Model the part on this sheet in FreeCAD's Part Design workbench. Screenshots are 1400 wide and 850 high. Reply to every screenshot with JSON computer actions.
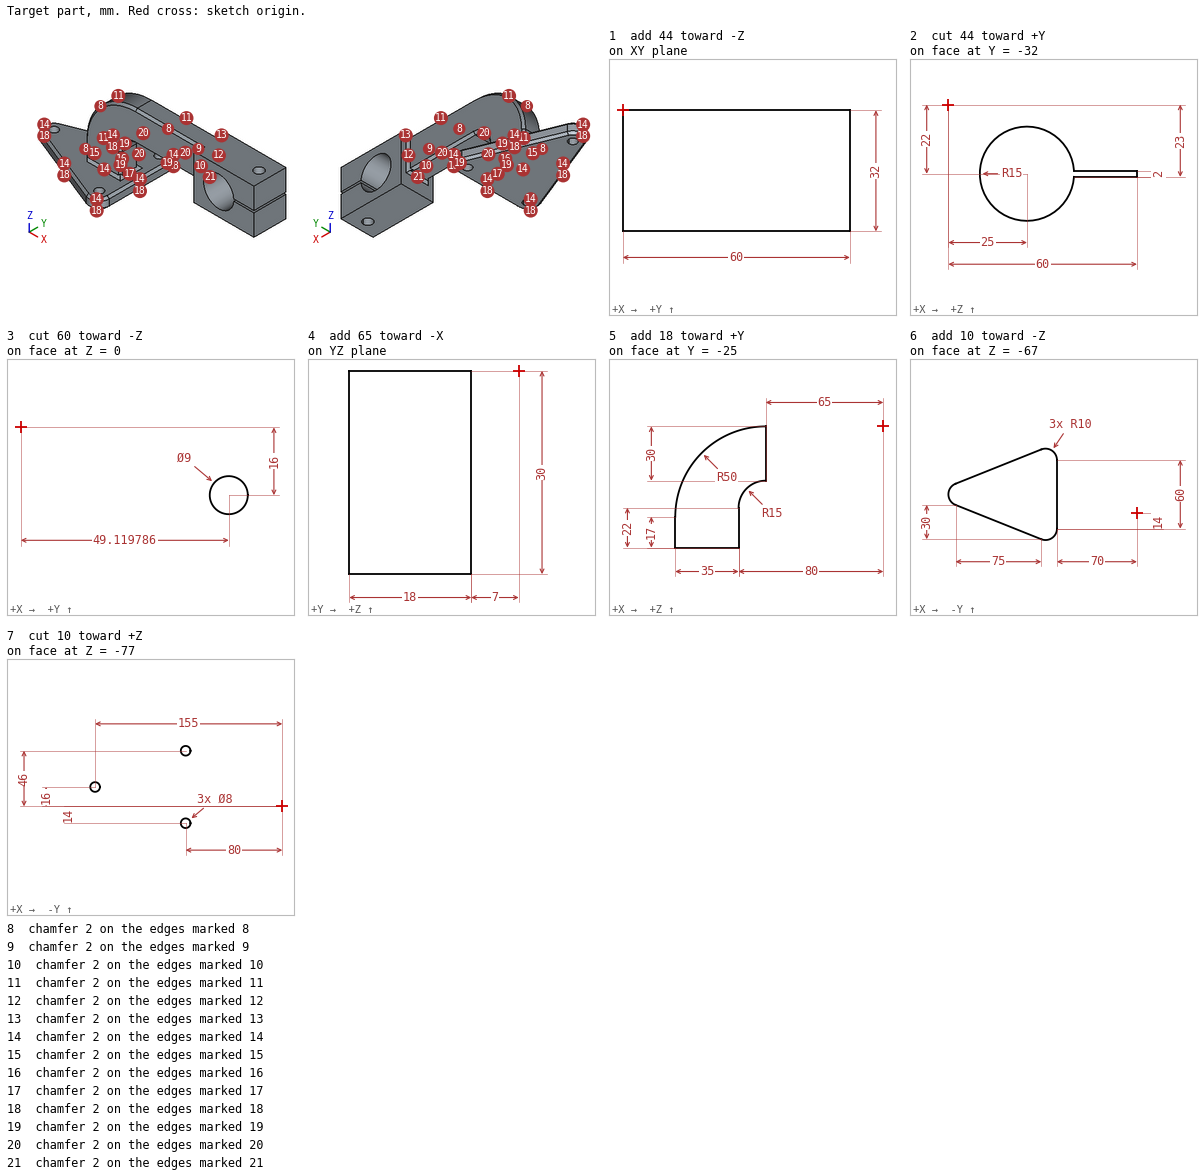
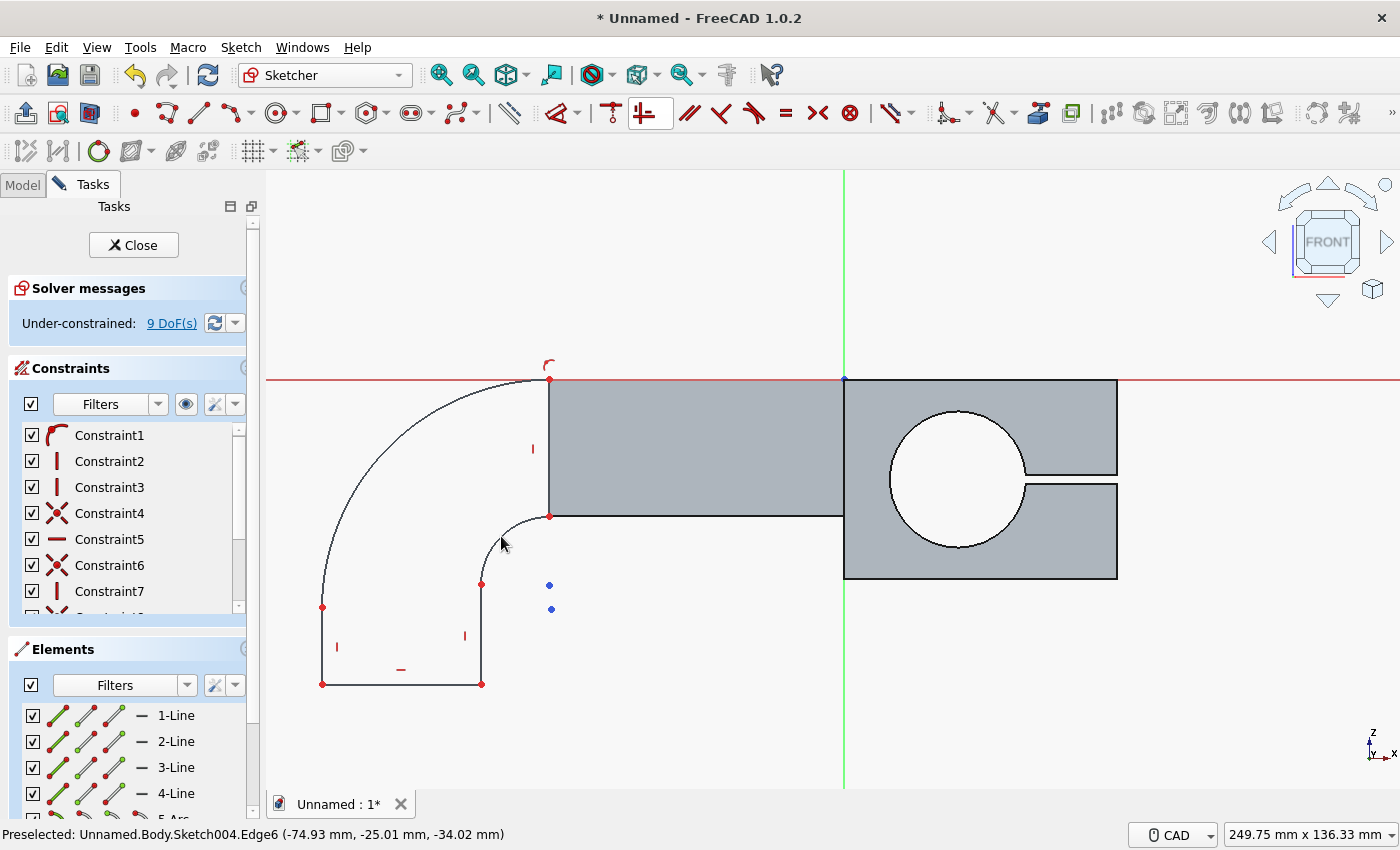
{"action": "left_click", "coordinate": [481, 655]}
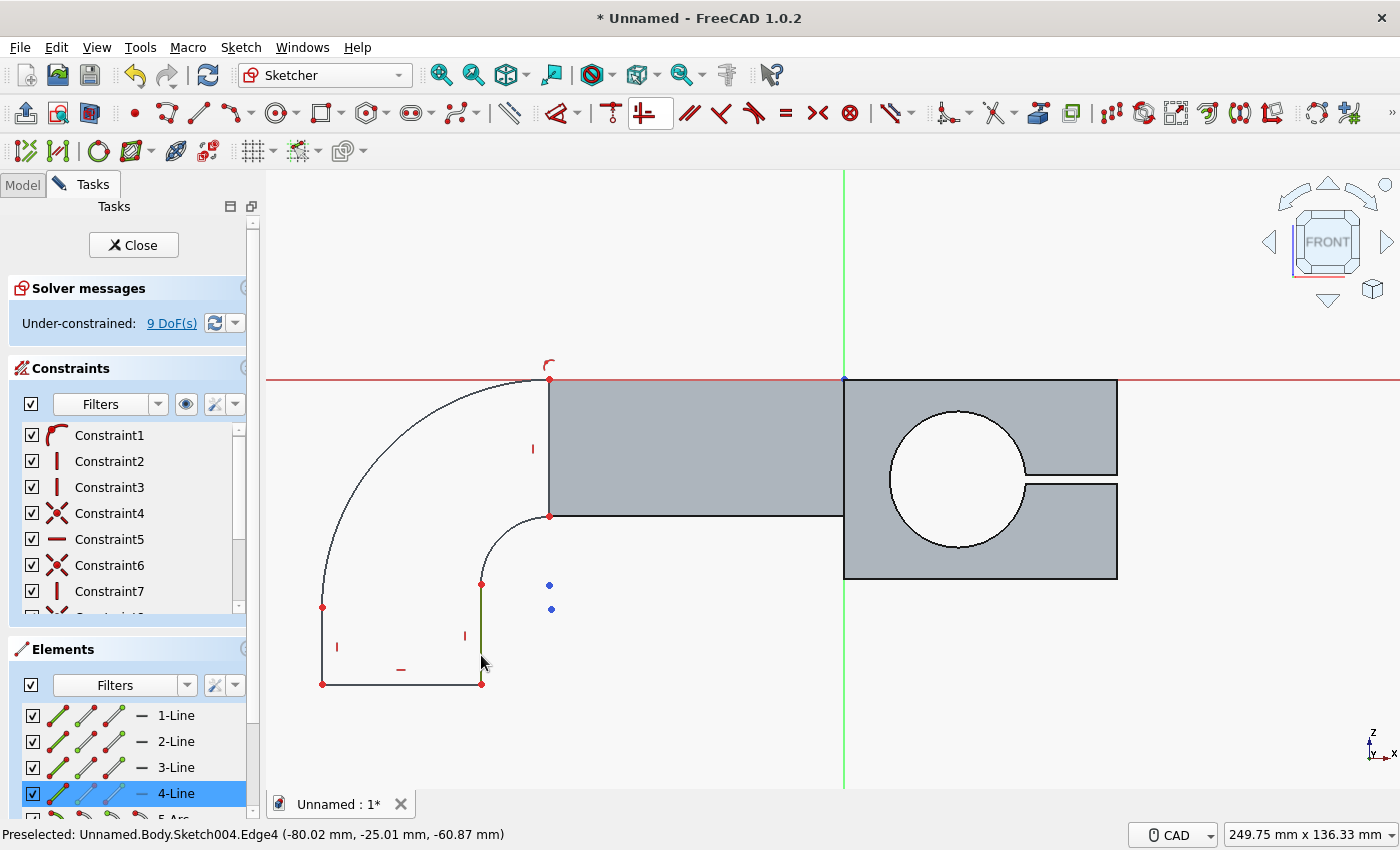
{"action": "left_click", "coordinate": [518, 524]}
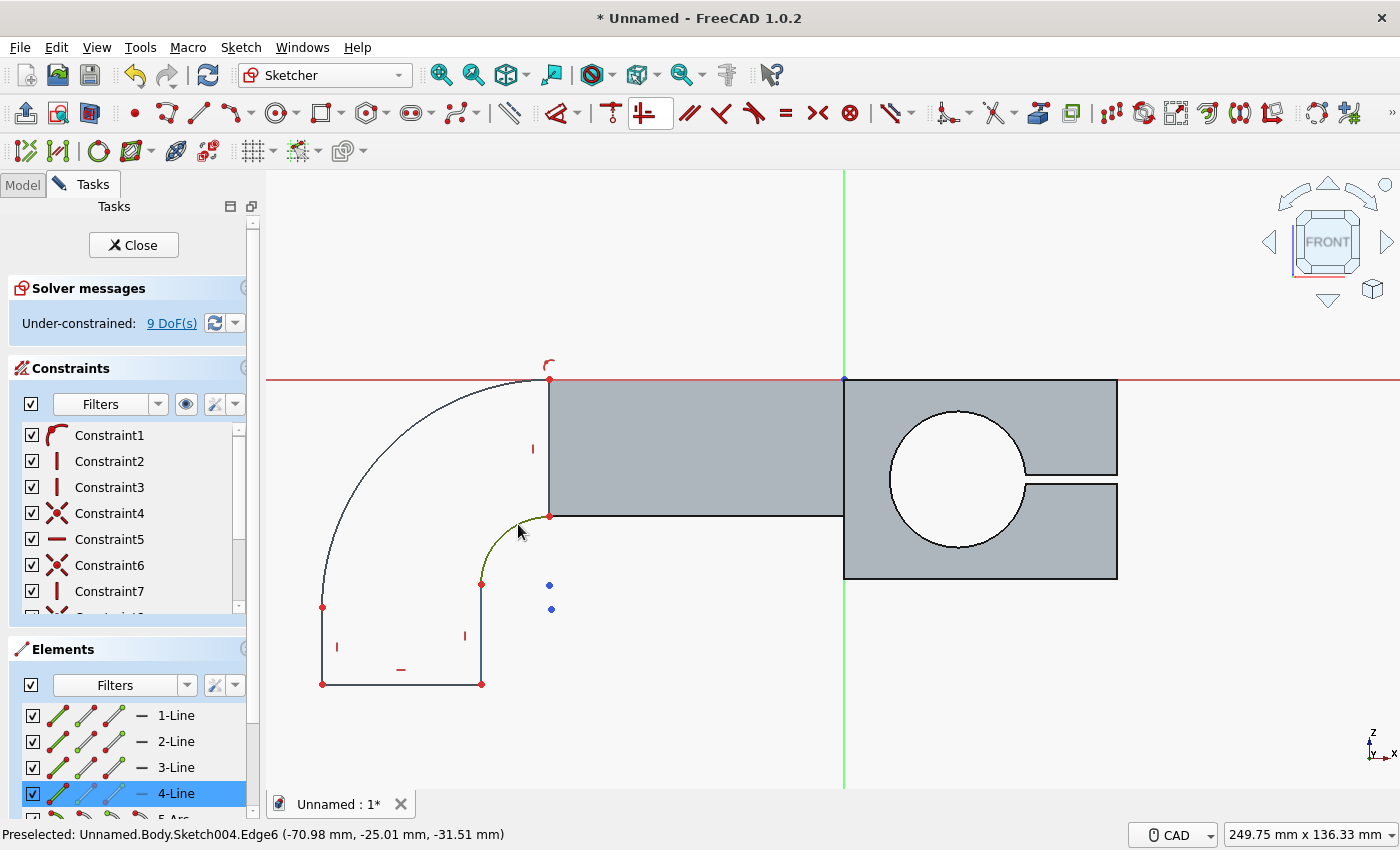
{"action": "left_click", "coordinate": [754, 114]}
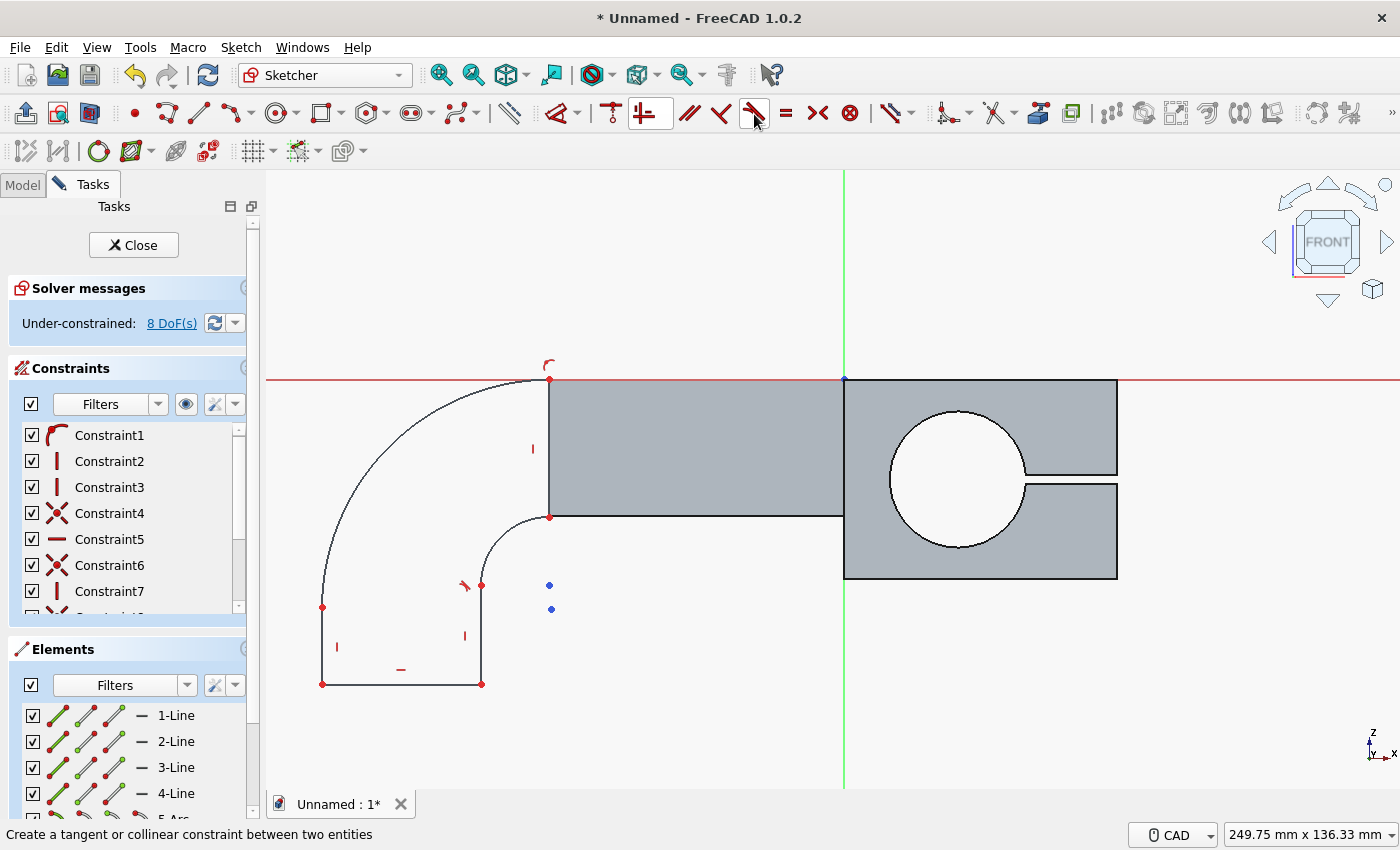
{"action": "left_click", "coordinate": [556, 114]}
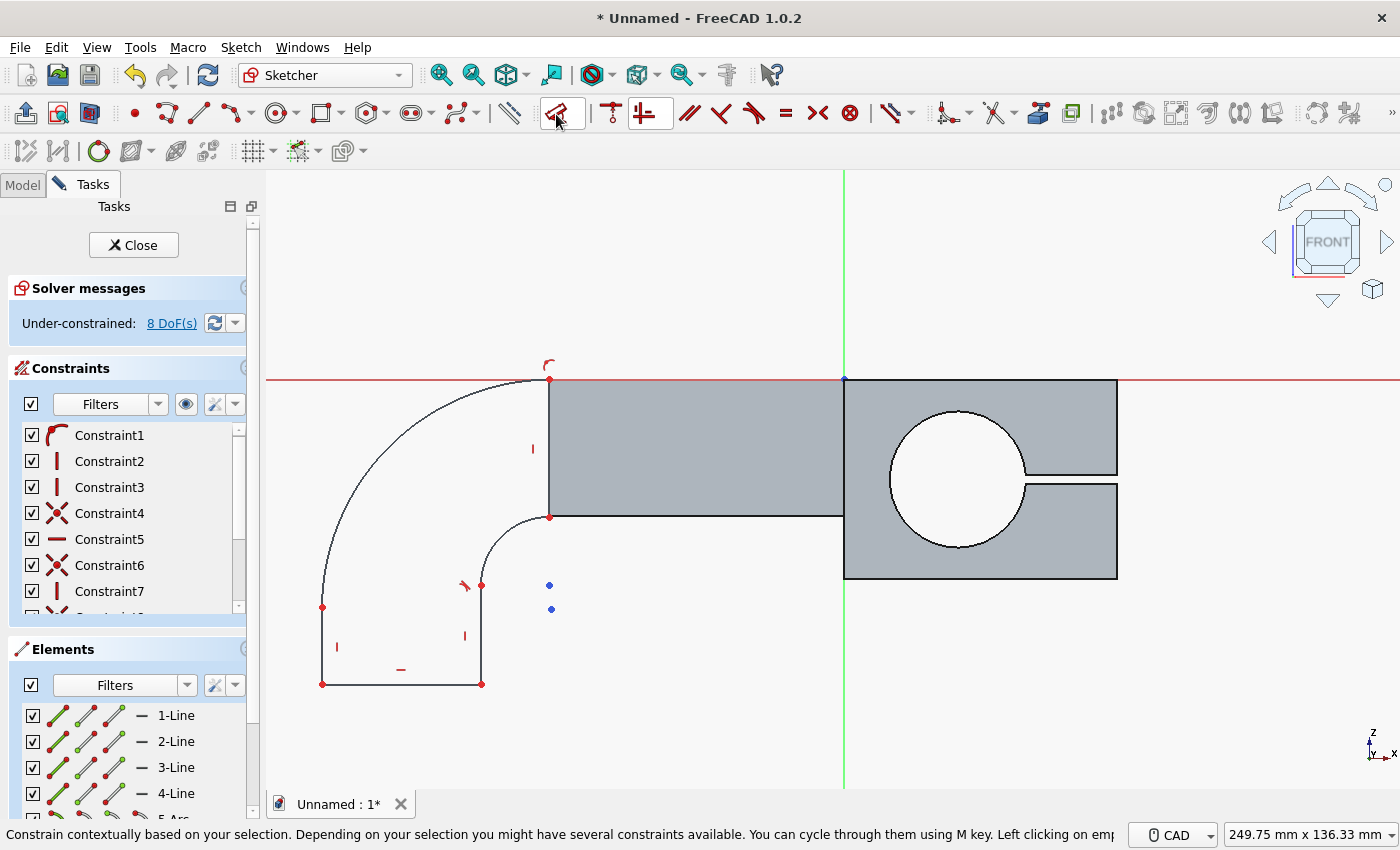
{"action": "left_click", "coordinate": [446, 405]}
{"action": "left_click", "coordinate": [557, 347]}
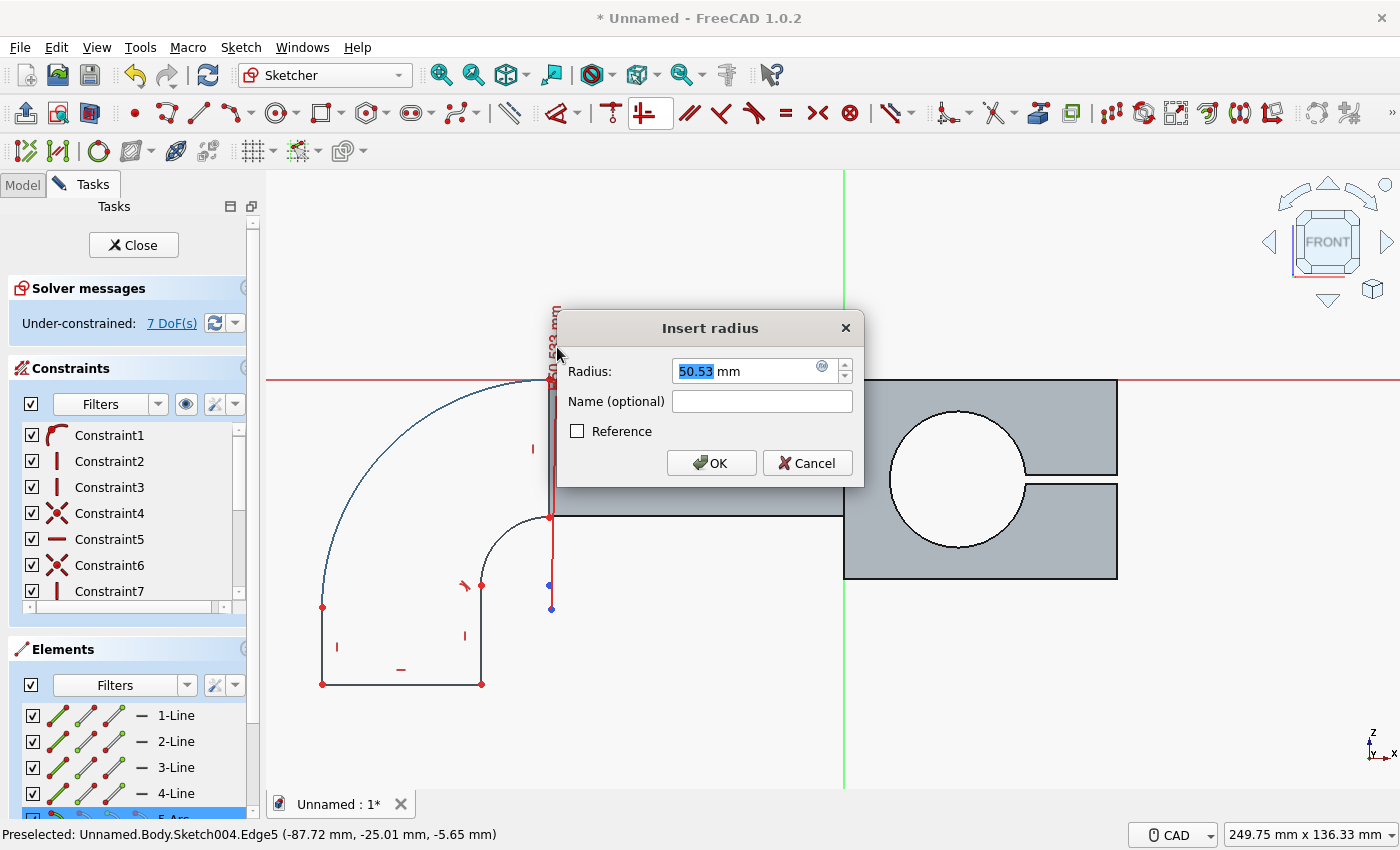
{"action": "type", "text": "50"}
{"action": "key", "text": "Return"}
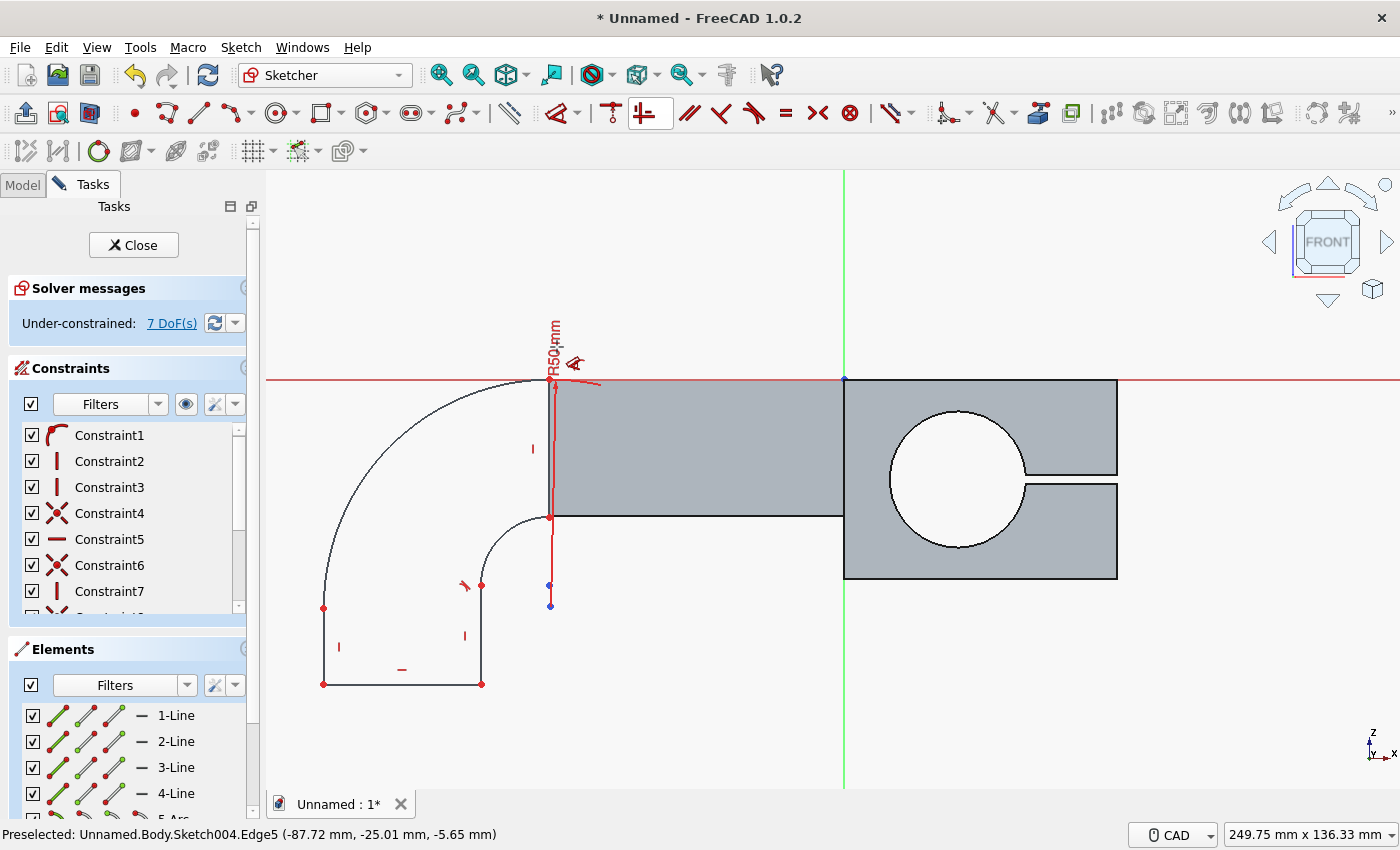
{"action": "left_click", "coordinate": [518, 525]}
{"action": "left_click", "coordinate": [503, 497]}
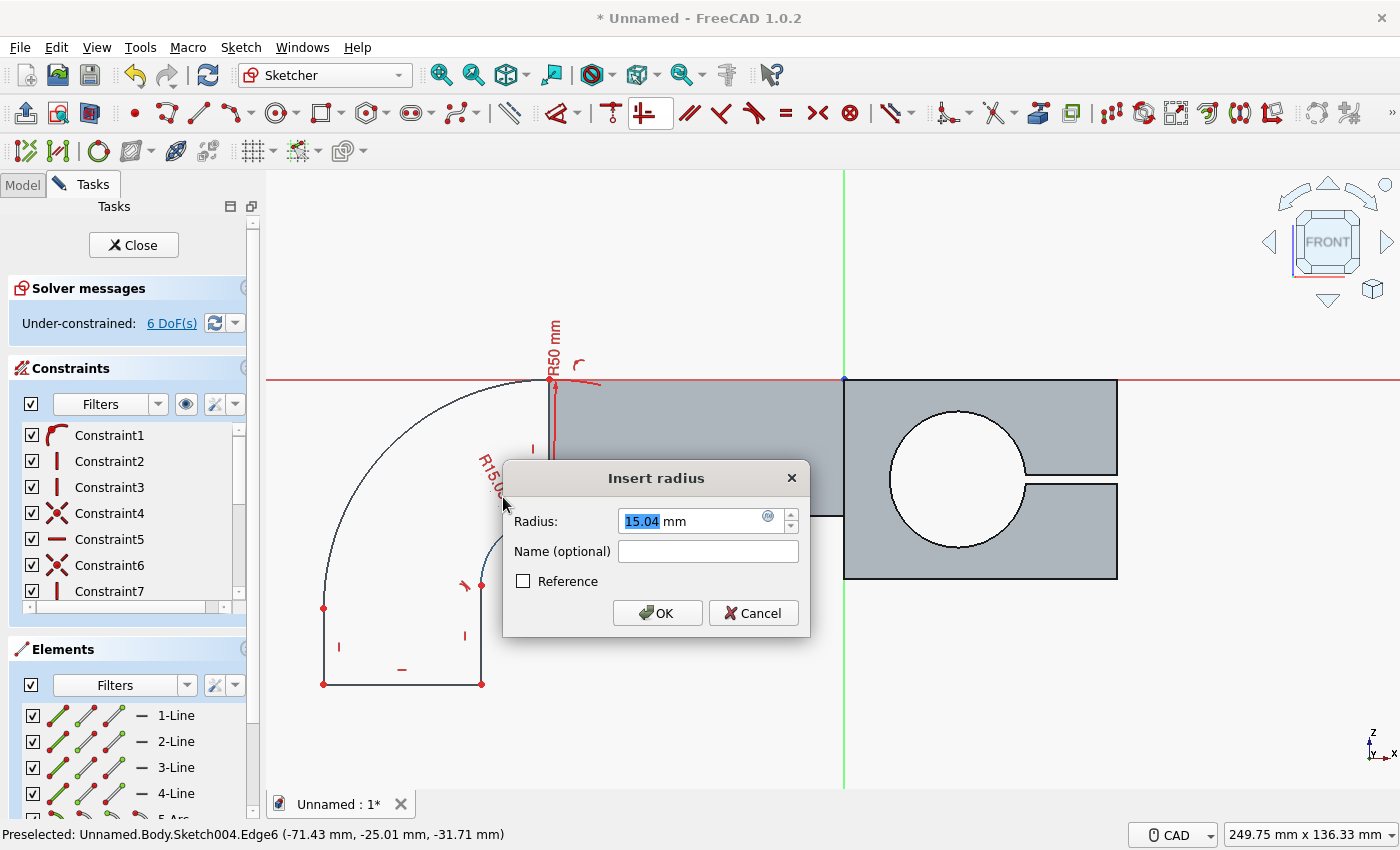
{"action": "type", "text": "15"}
{"action": "key", "text": "Return"}